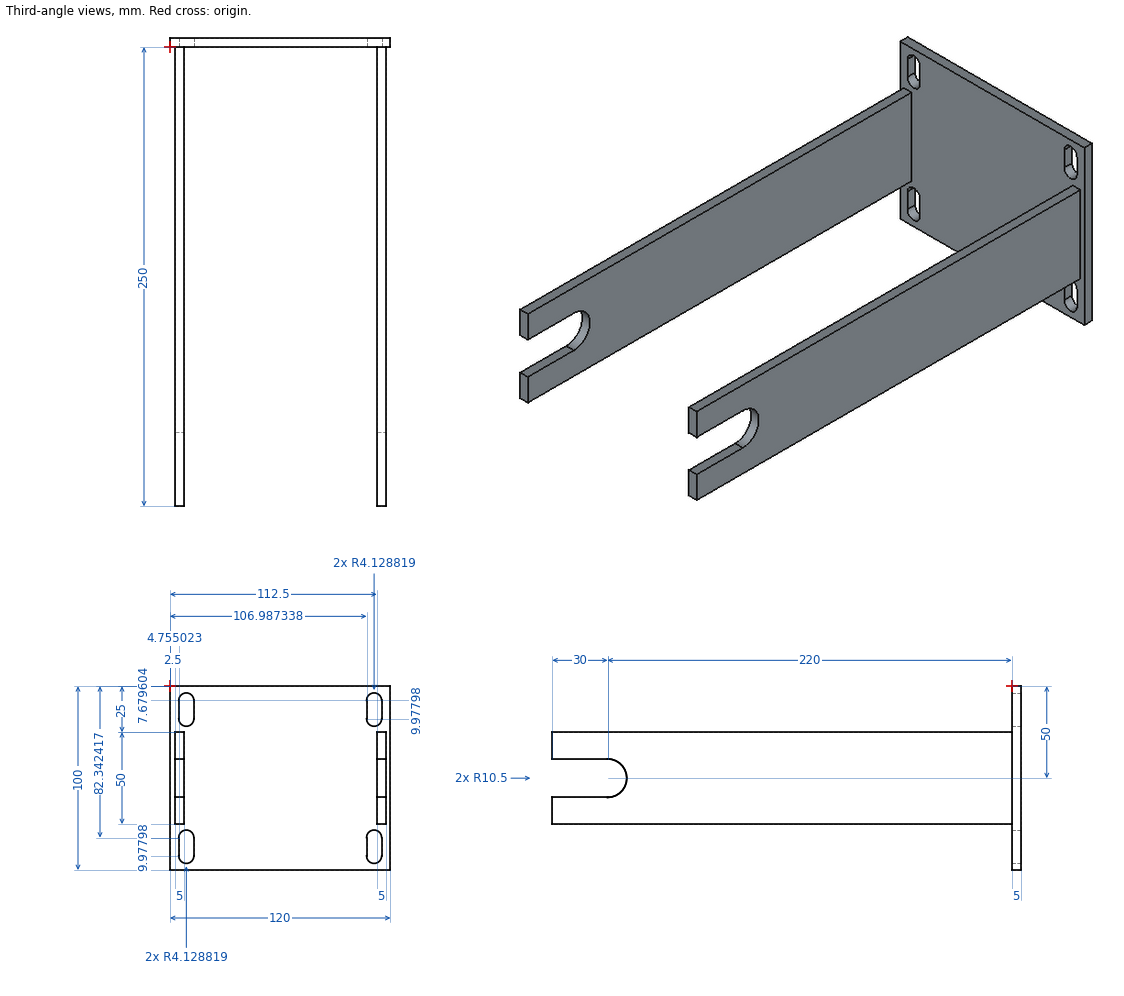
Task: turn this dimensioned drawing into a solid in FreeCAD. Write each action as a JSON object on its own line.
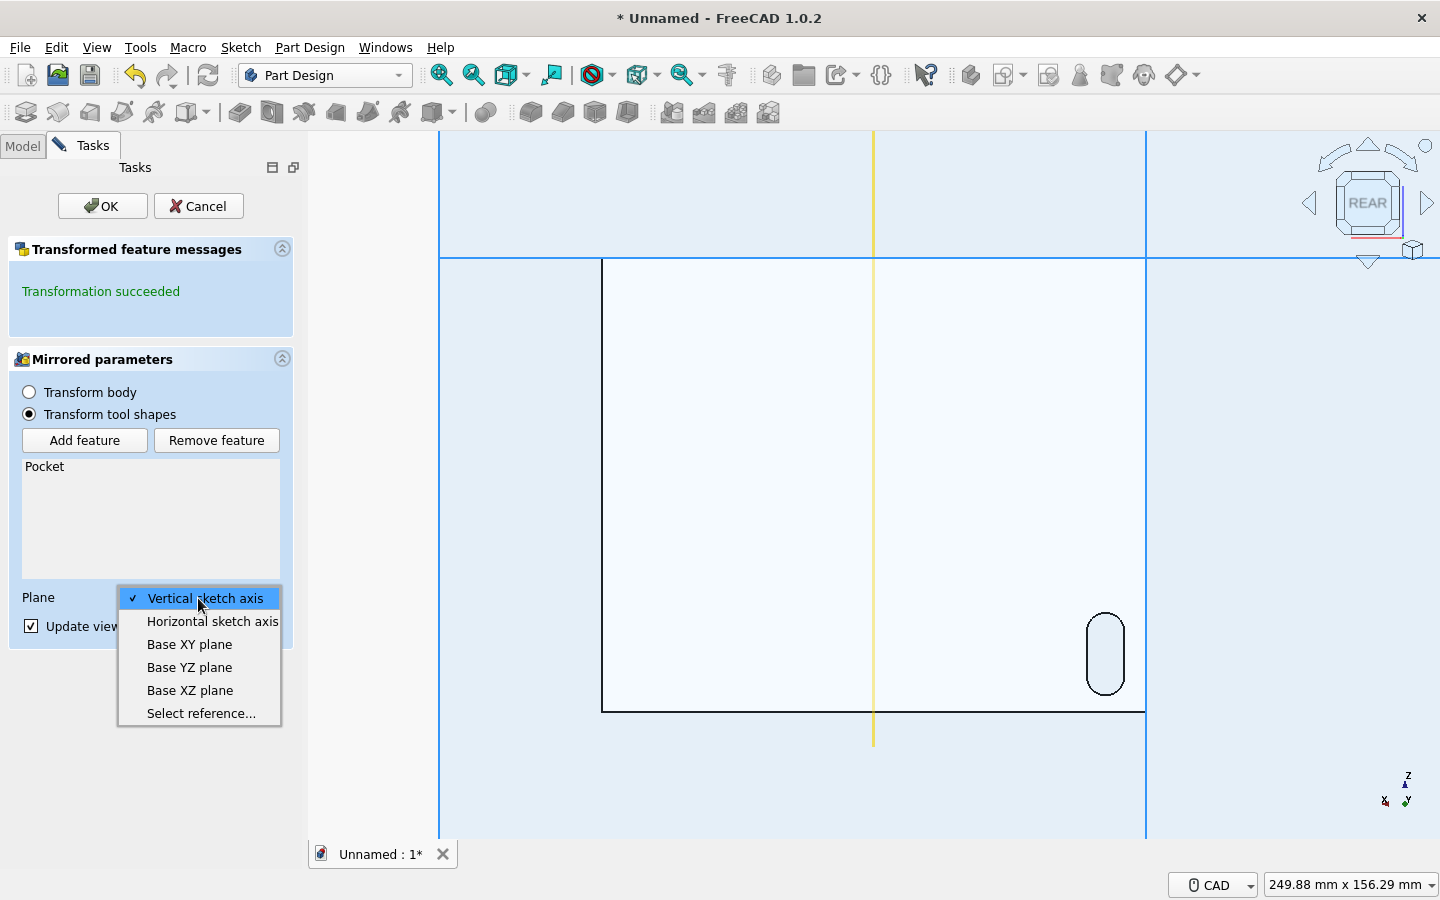
{"action": "left_click", "coordinate": [198, 714]}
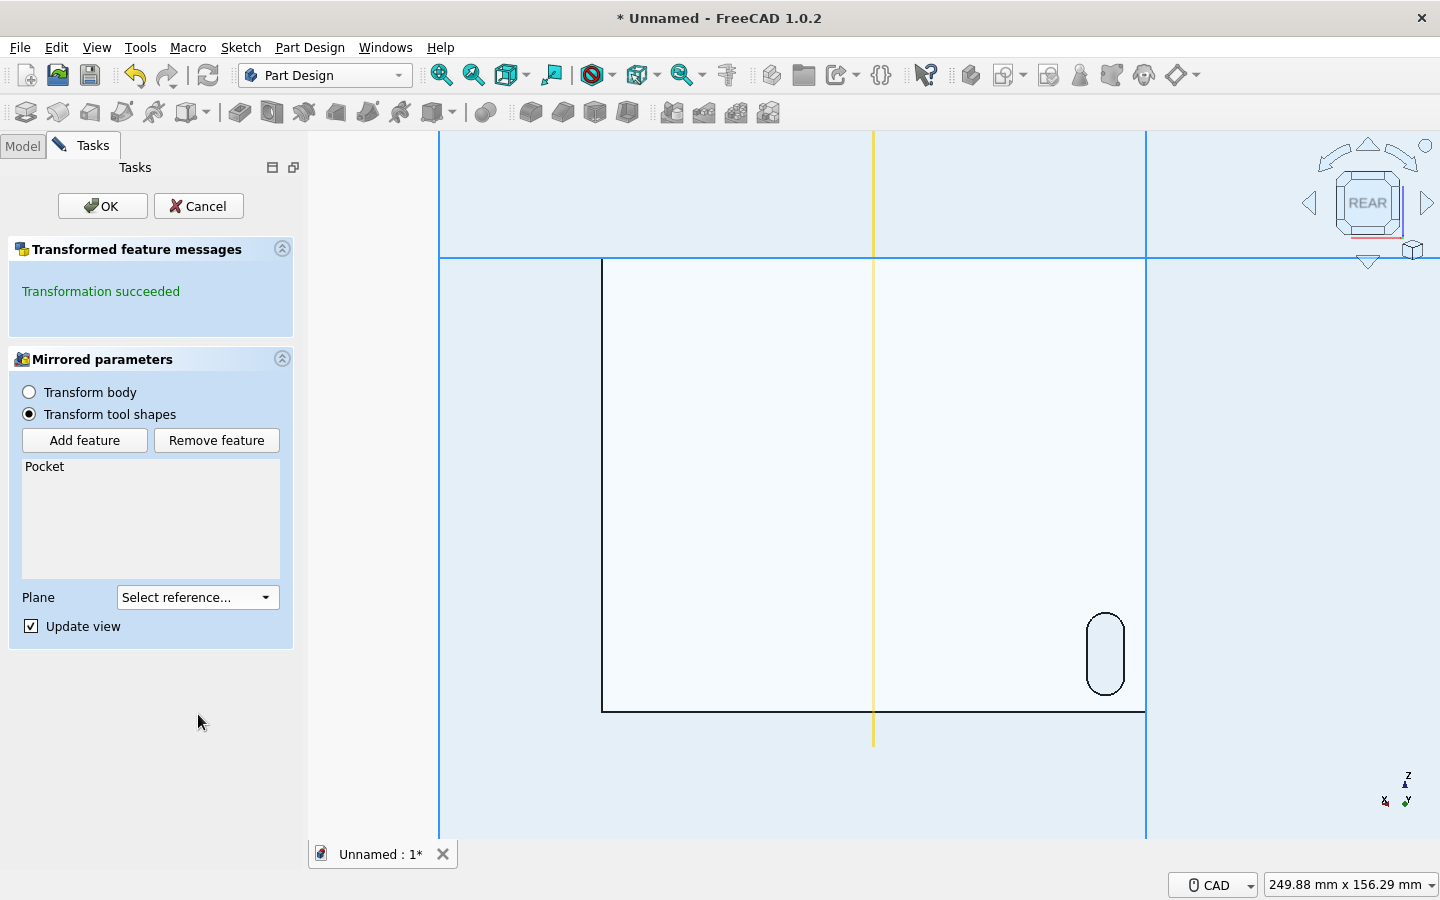
{"action": "left_click", "coordinate": [23, 145]}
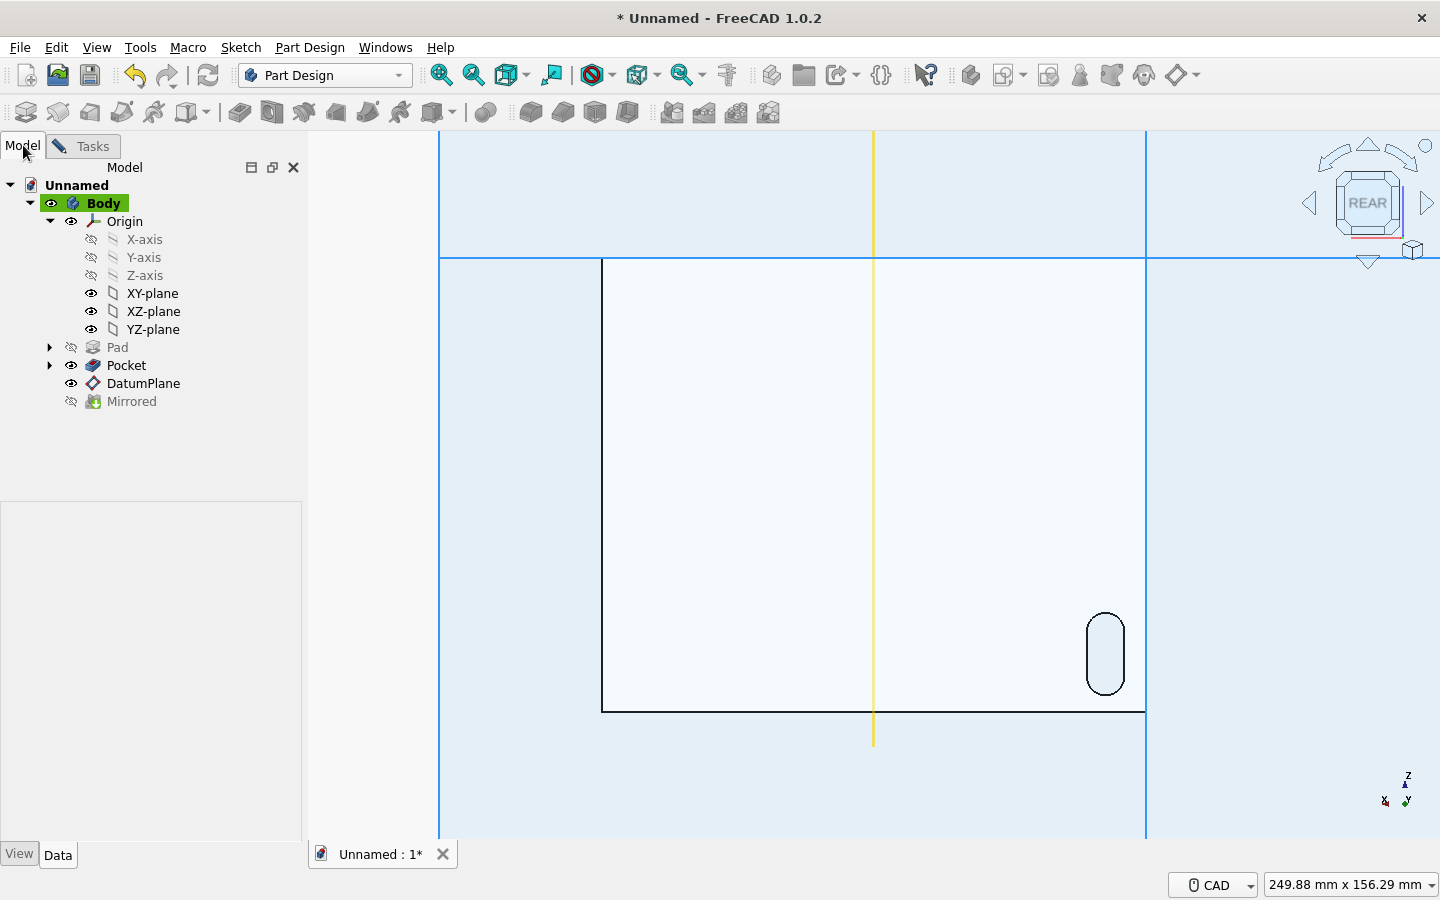
{"action": "left_click", "coordinate": [116, 383]}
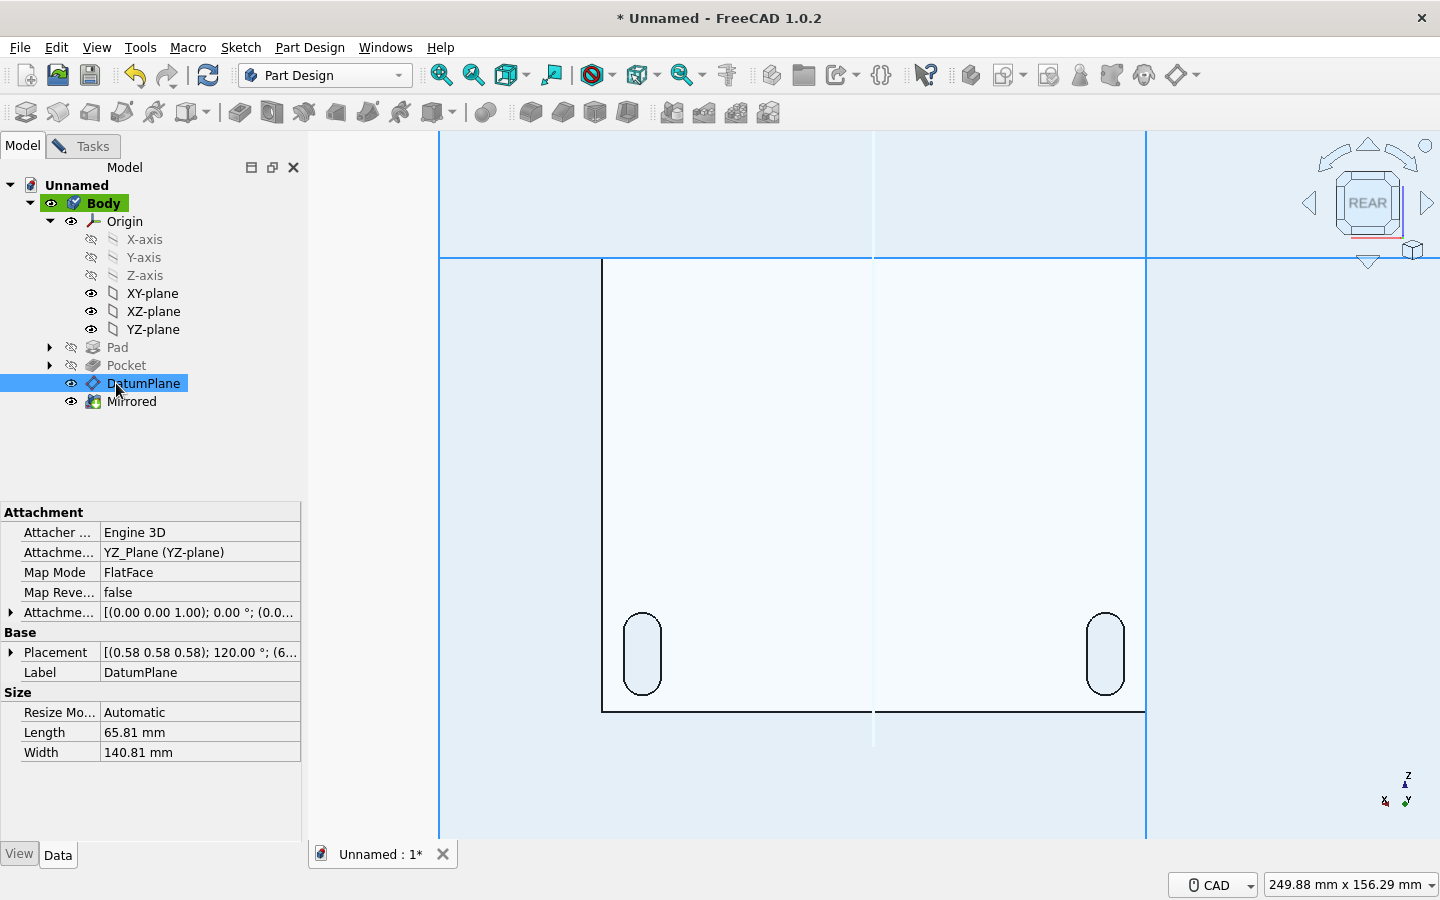
{"action": "left_click", "coordinate": [84, 145]}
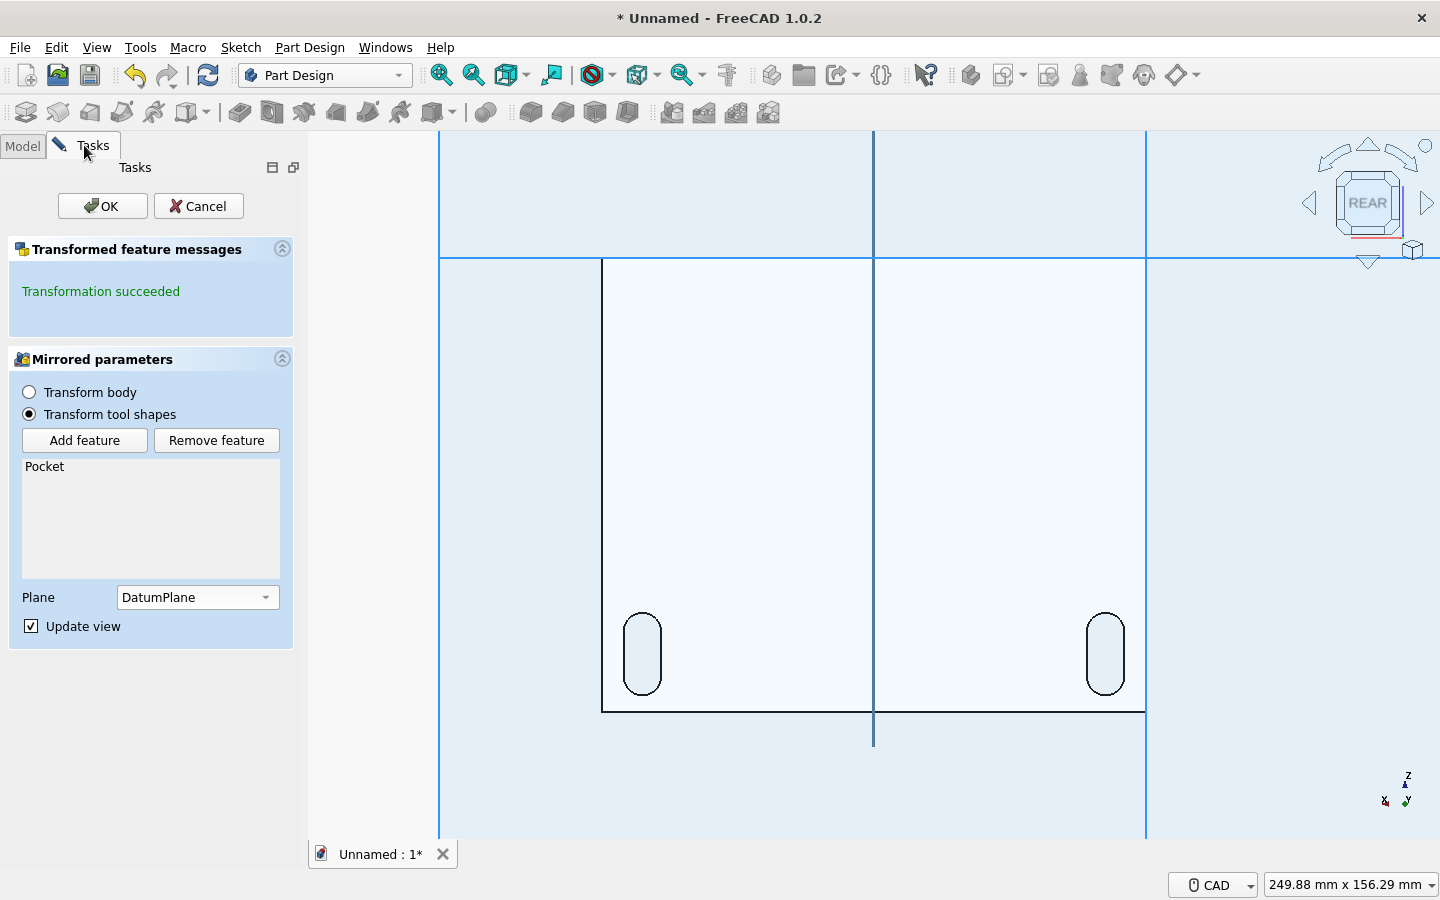
{"action": "left_click", "coordinate": [103, 206]}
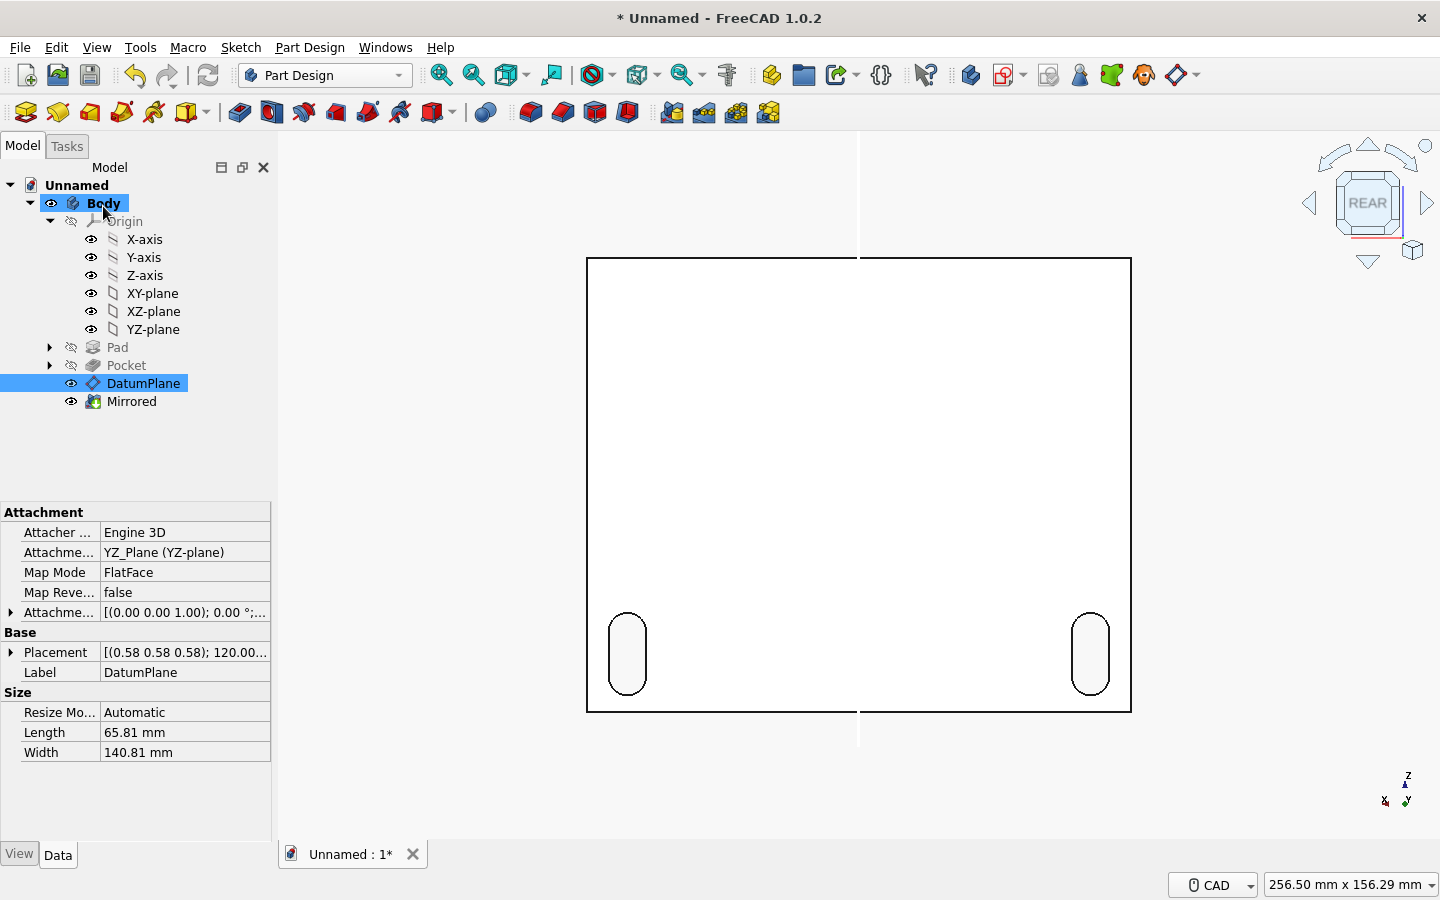
{"action": "left_click", "coordinate": [116, 383]}
{"action": "key", "text": "space"}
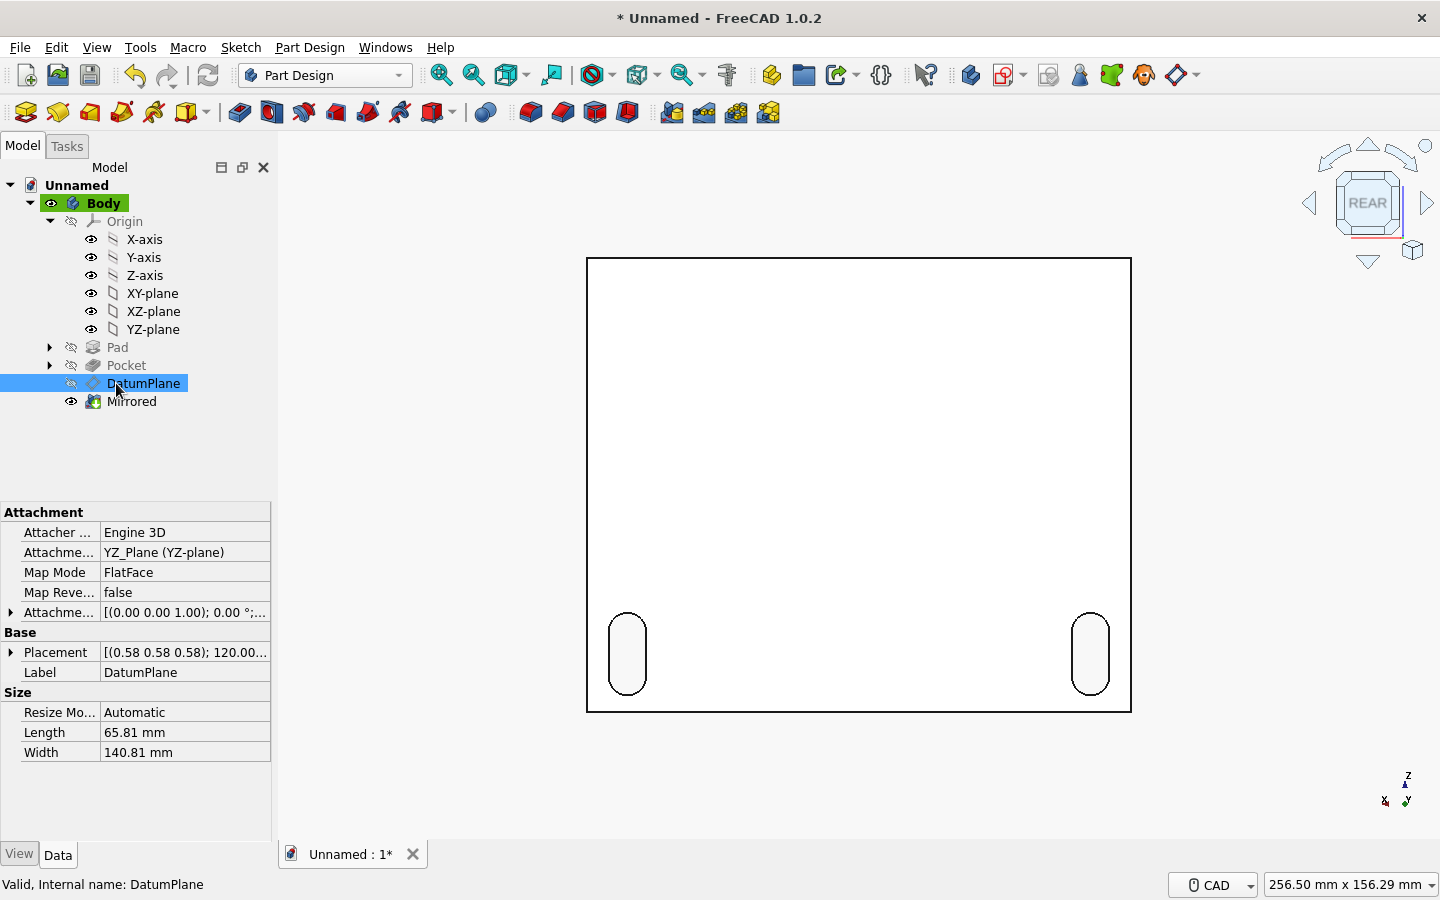
{"action": "left_click", "coordinate": [136, 293]}